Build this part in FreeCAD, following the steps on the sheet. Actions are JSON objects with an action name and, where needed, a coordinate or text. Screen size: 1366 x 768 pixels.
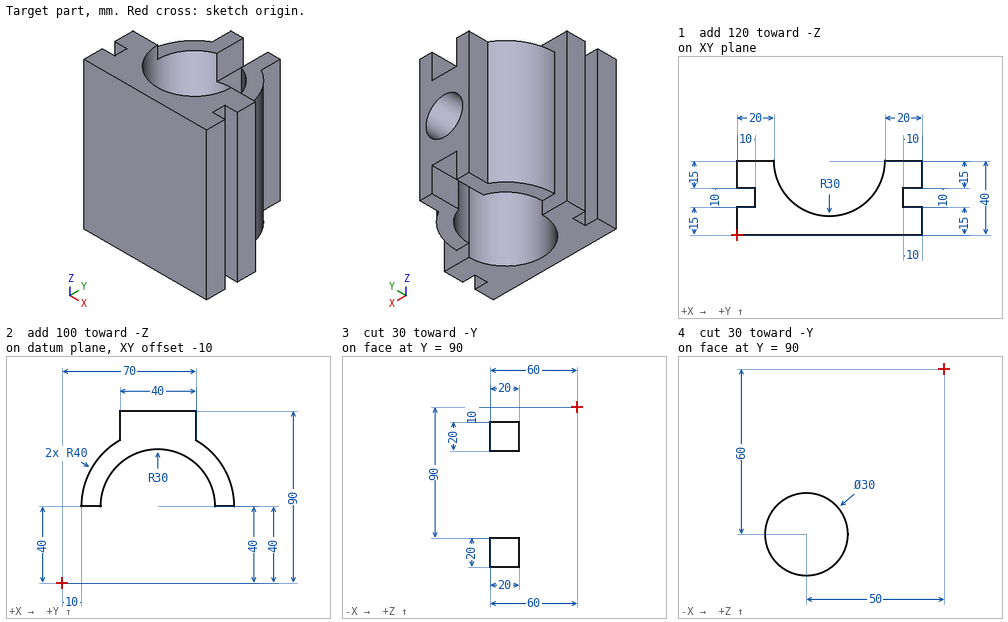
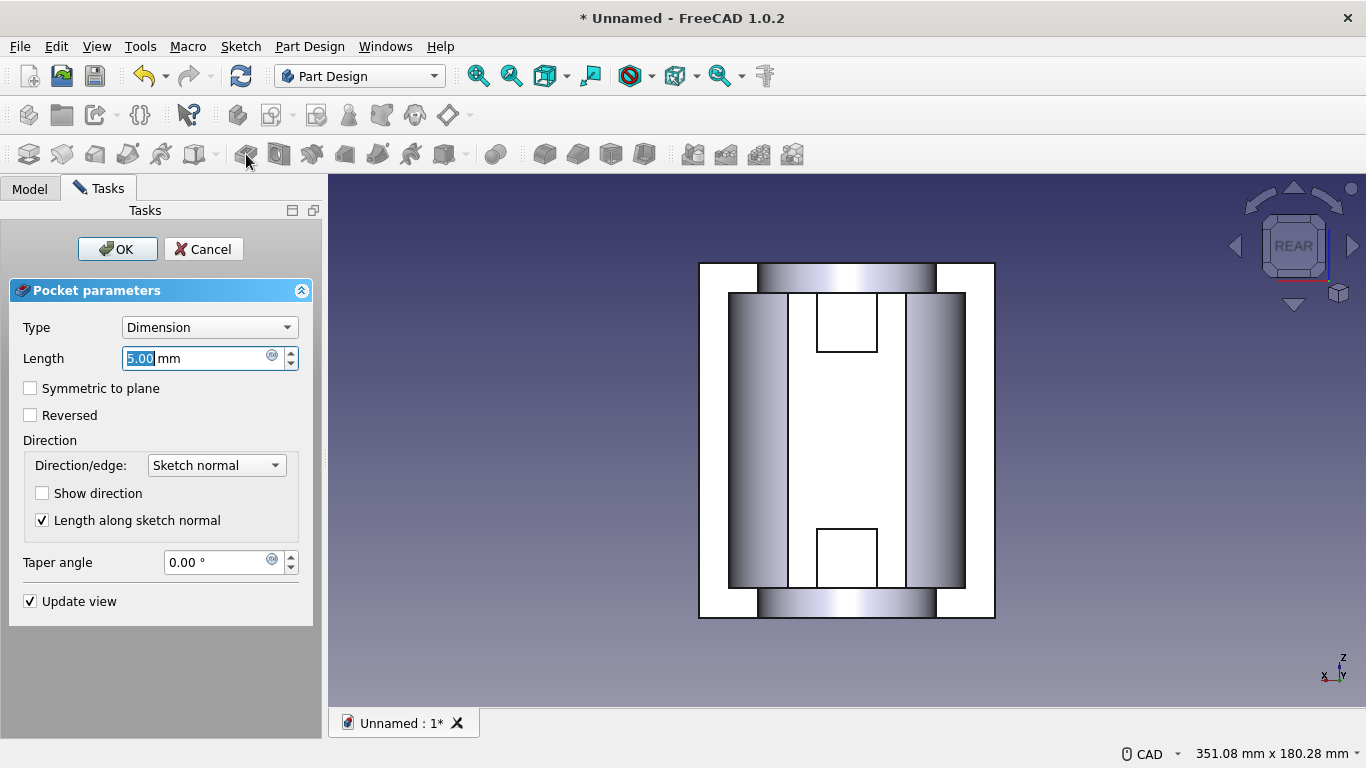
{"action": "type", "text": "30"}
{"action": "key", "text": "Tab"}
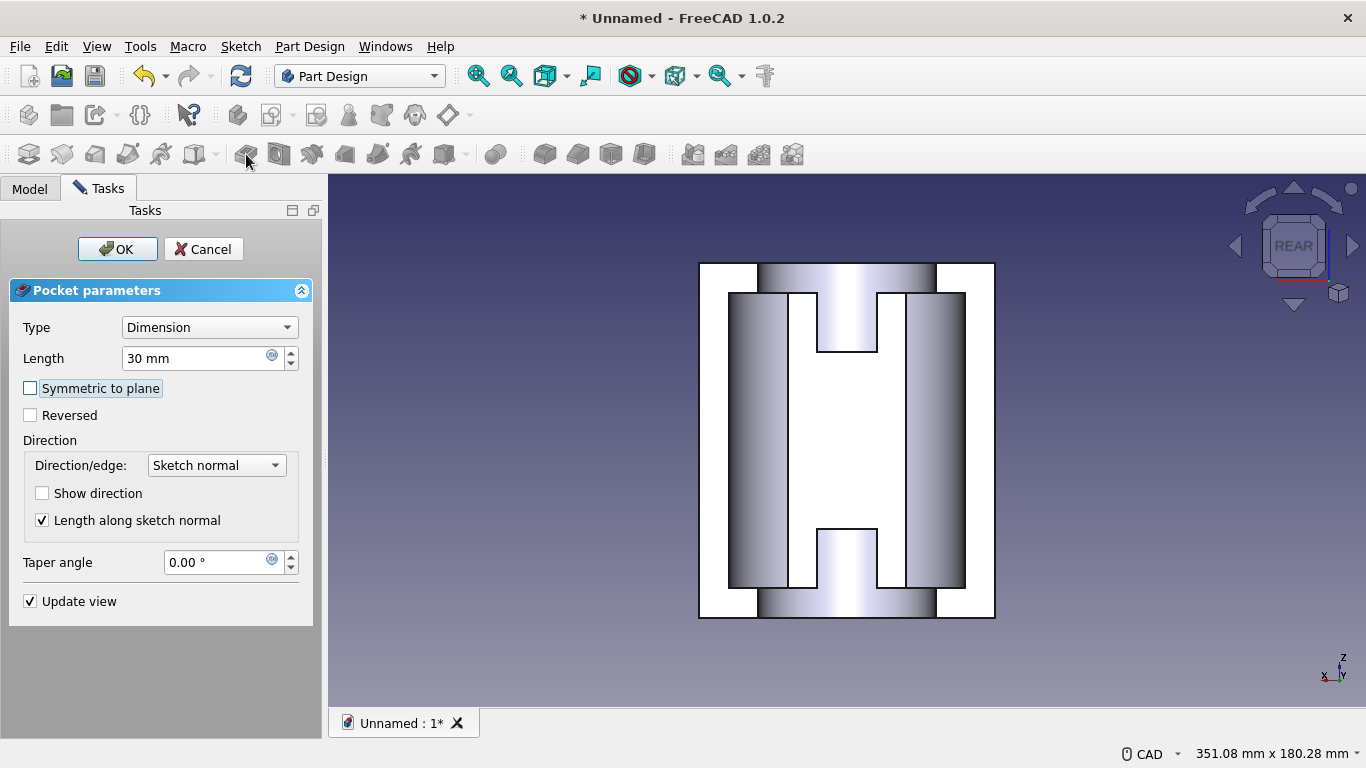
{"action": "left_click", "coordinate": [118, 249]}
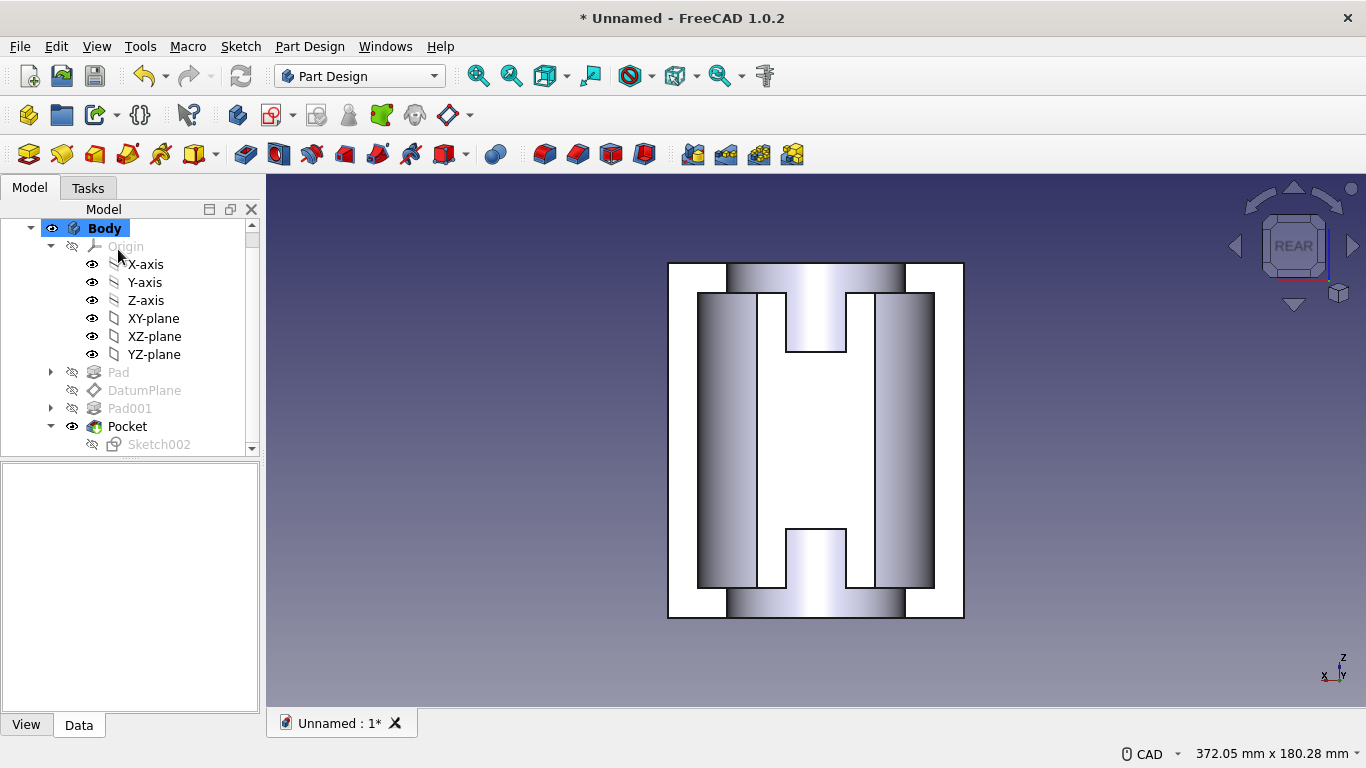
{"action": "left_click", "coordinate": [816, 440]}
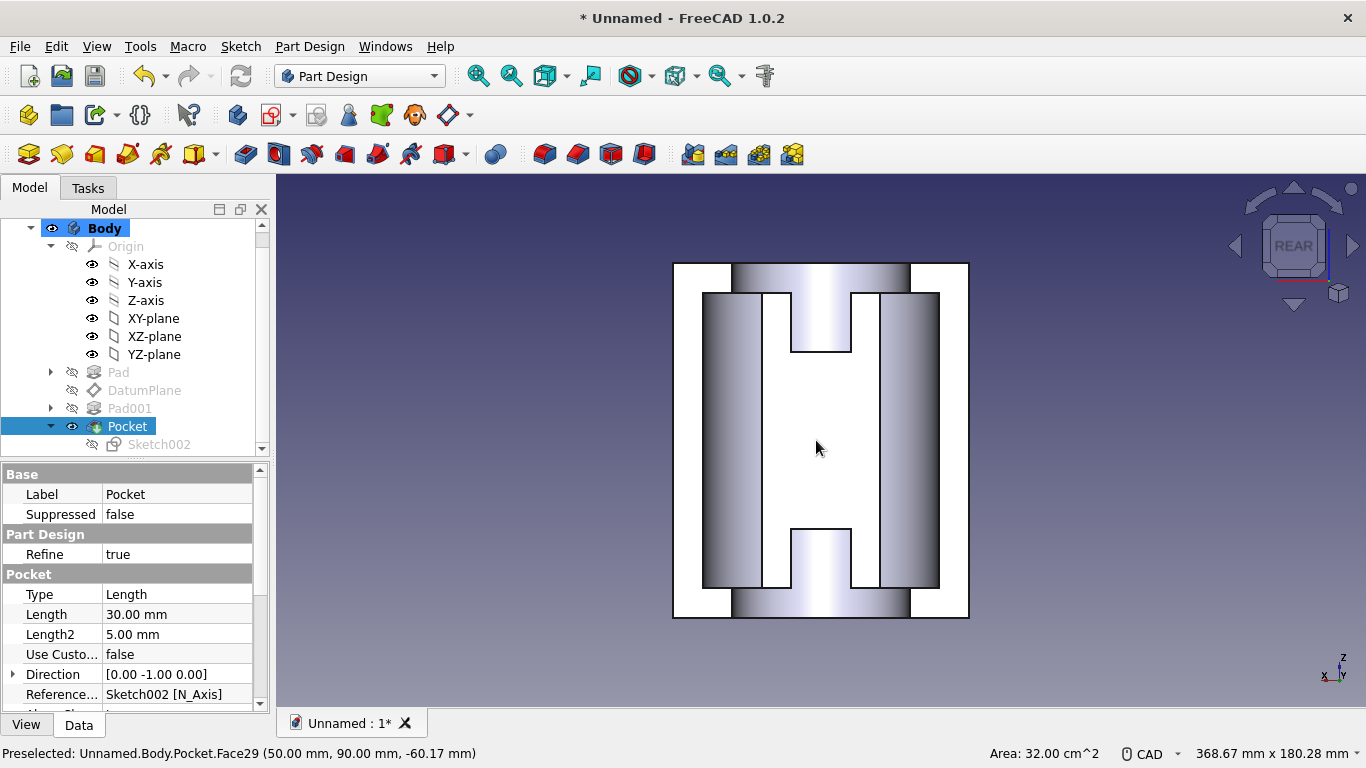
{"action": "left_click", "coordinate": [270, 116]}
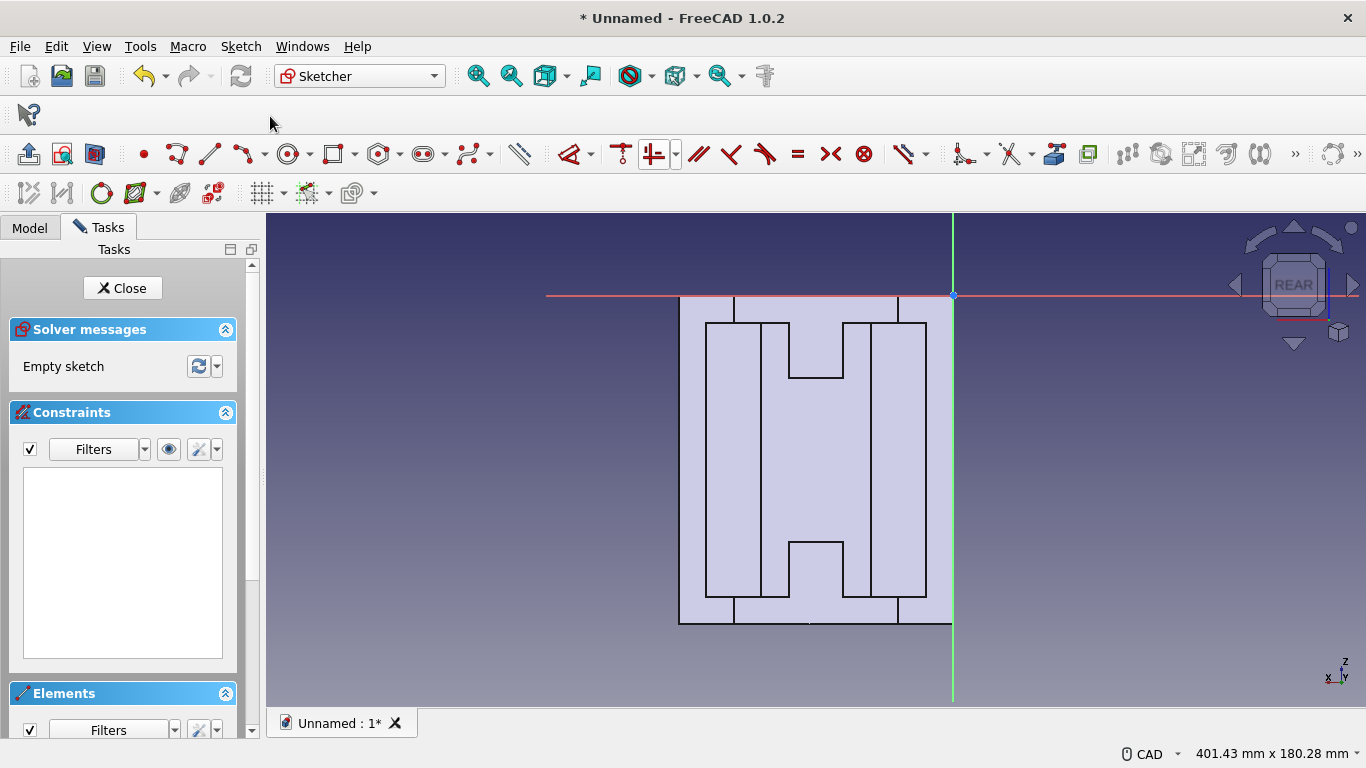
{"action": "scroll", "coordinate": [838, 460], "scroll_direction": "up", "scroll_amount": 7}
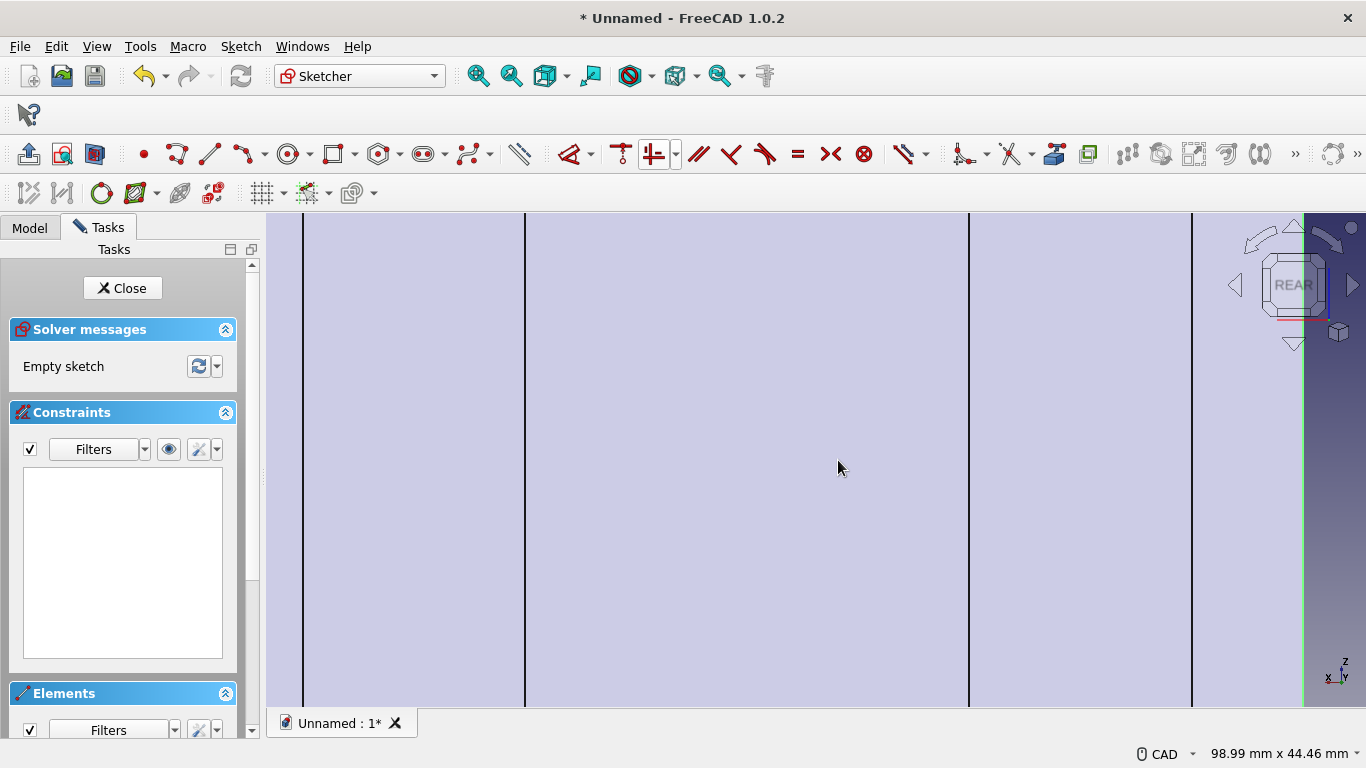
{"action": "left_click", "coordinate": [288, 154]}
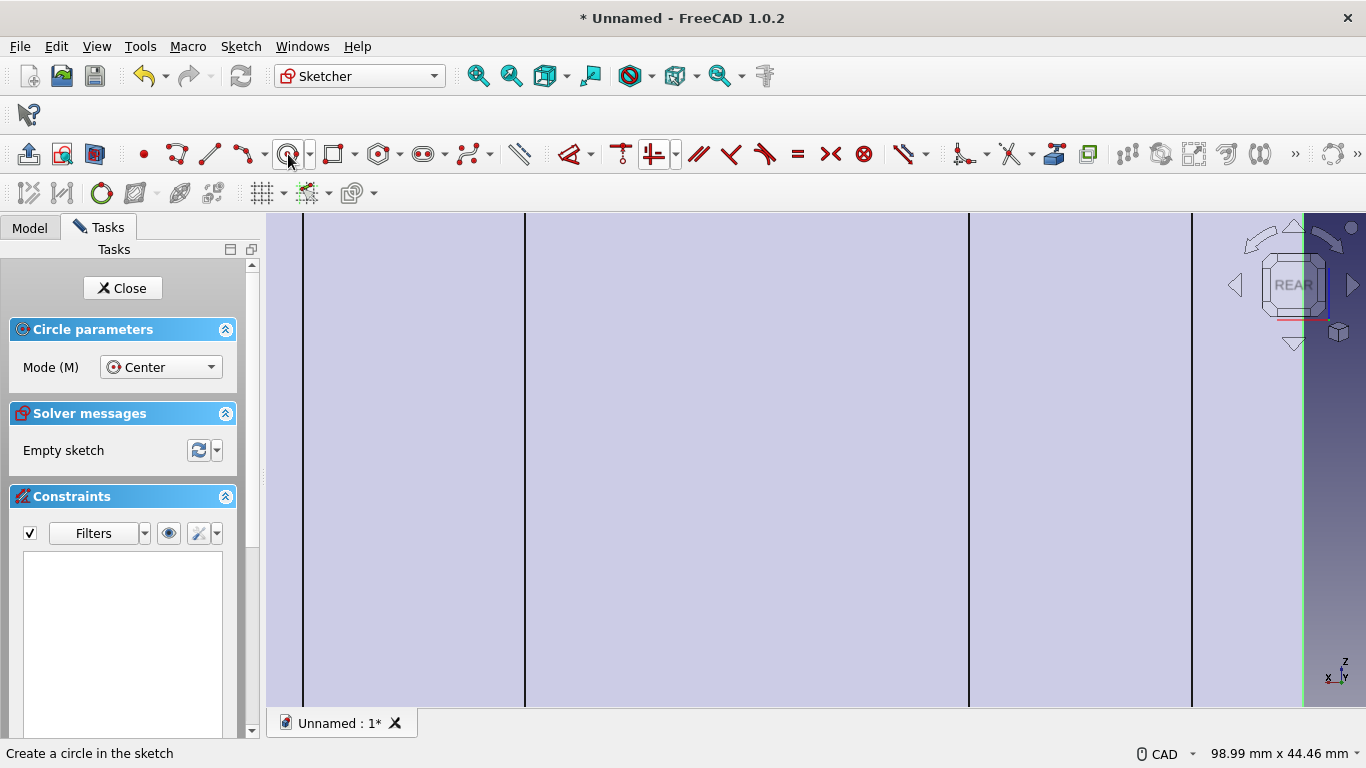
{"action": "left_click", "coordinate": [747, 458]}
{"action": "left_click", "coordinate": [865, 341]}
{"action": "key", "text": "Escape"}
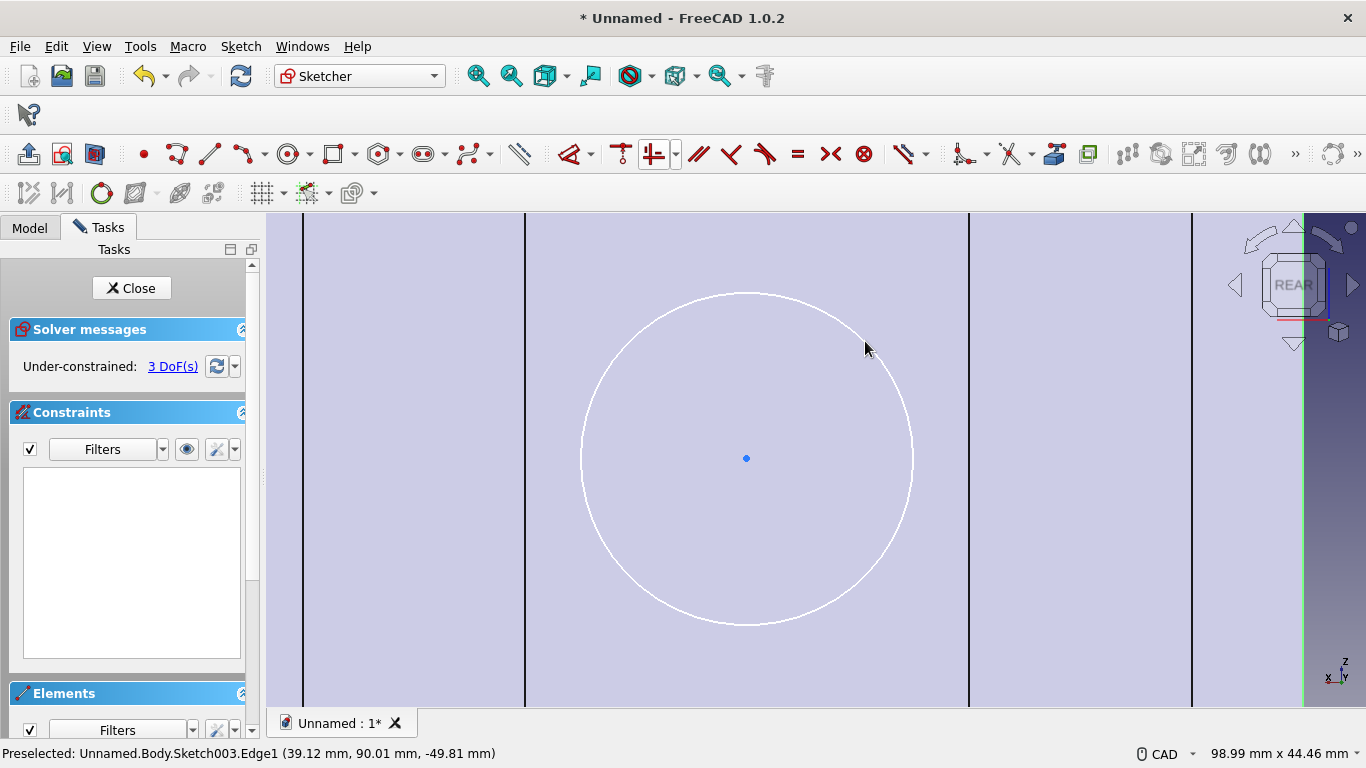
{"action": "left_click", "coordinate": [568, 154]}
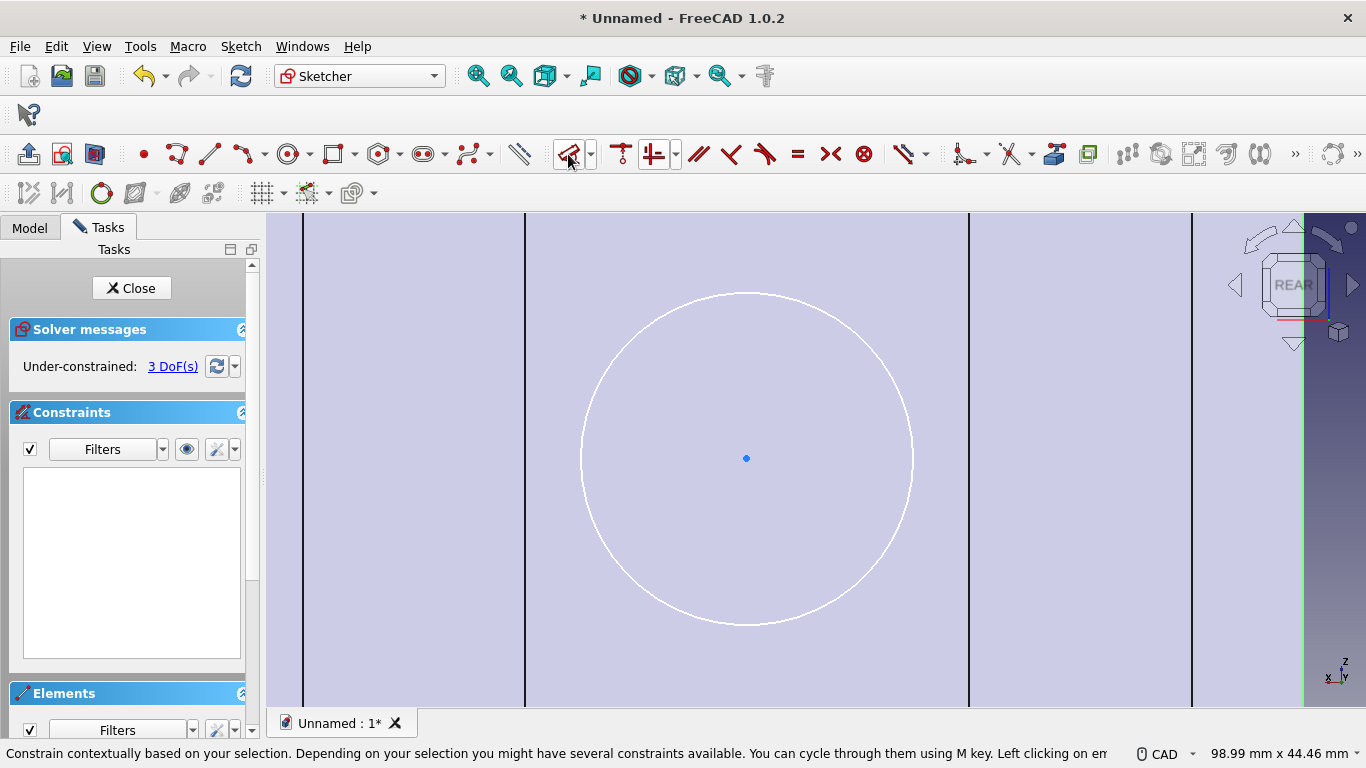
{"action": "left_click", "coordinate": [864, 341]}
{"action": "left_click", "coordinate": [887, 318]}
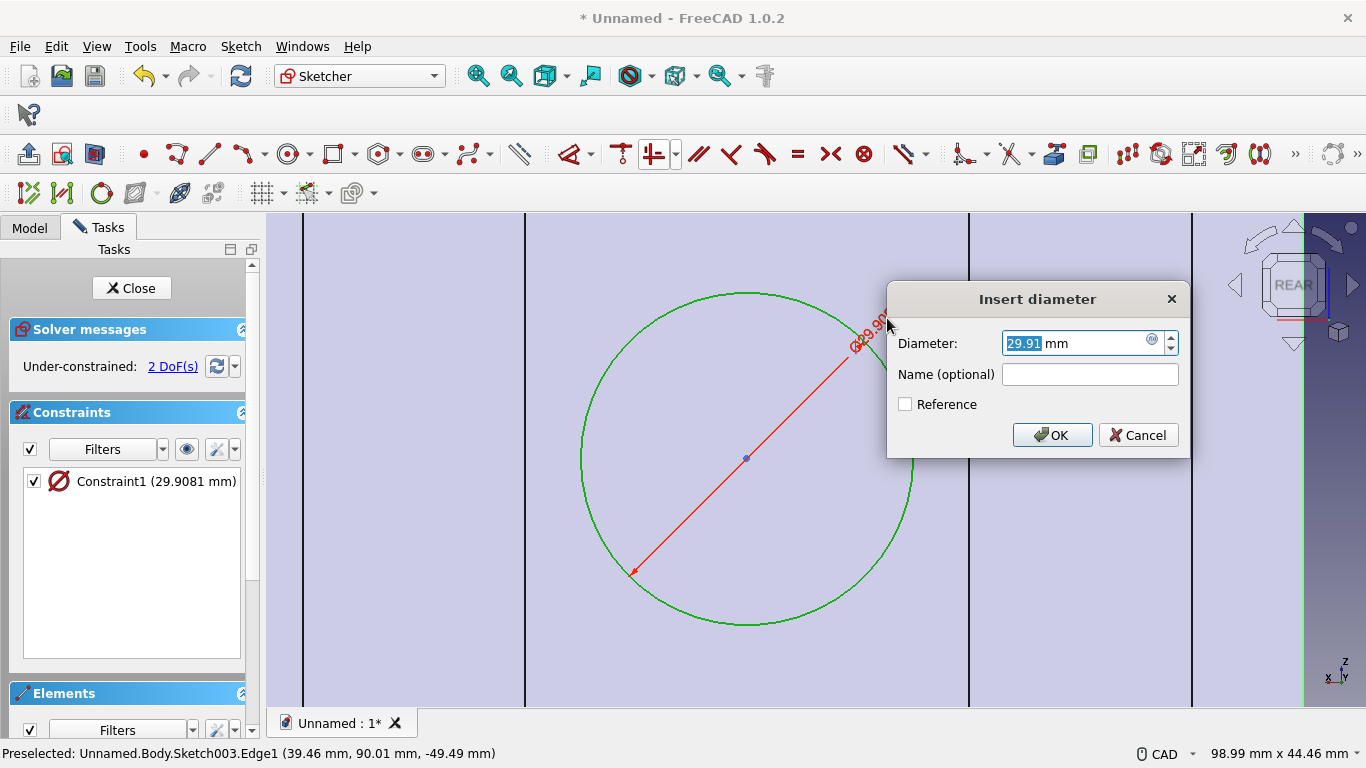
{"action": "type", "text": "30"}
{"action": "key", "text": "Return"}